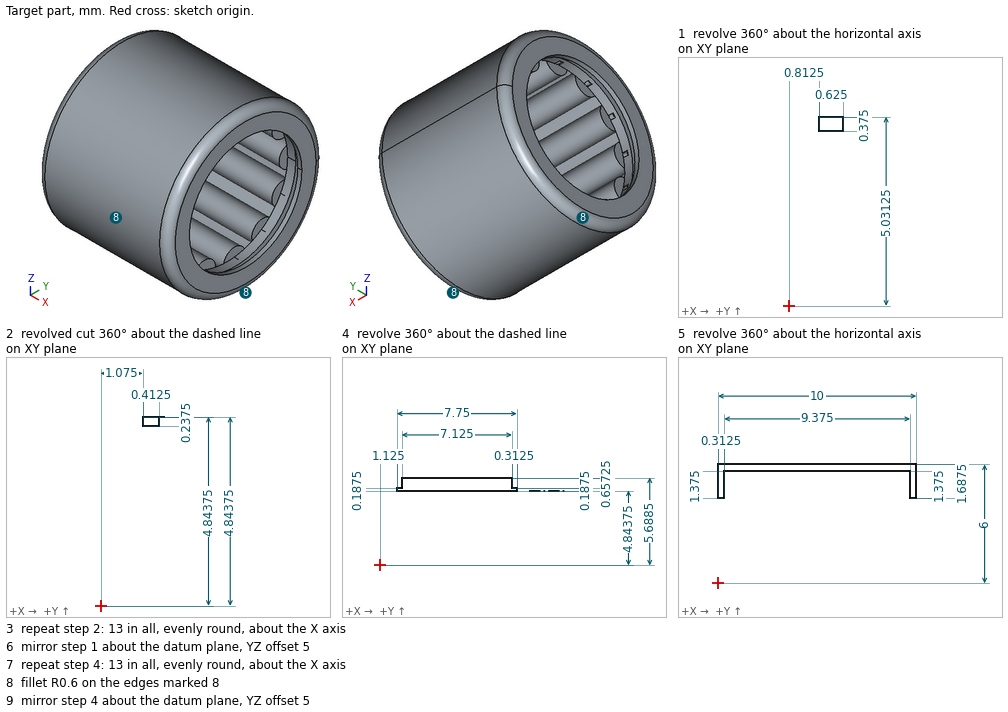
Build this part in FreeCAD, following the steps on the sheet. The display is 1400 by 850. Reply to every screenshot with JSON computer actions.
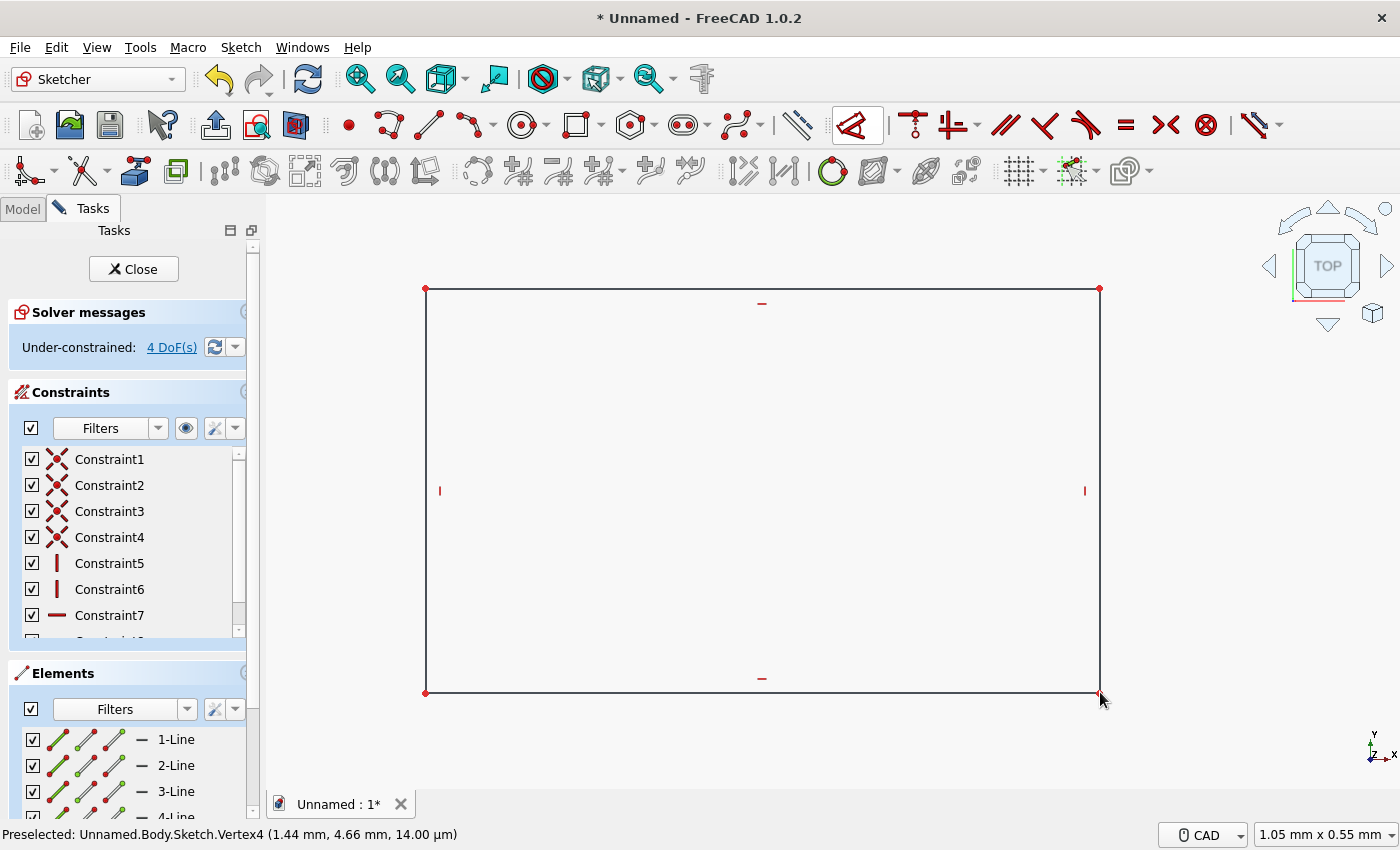
{"action": "key", "text": "d"}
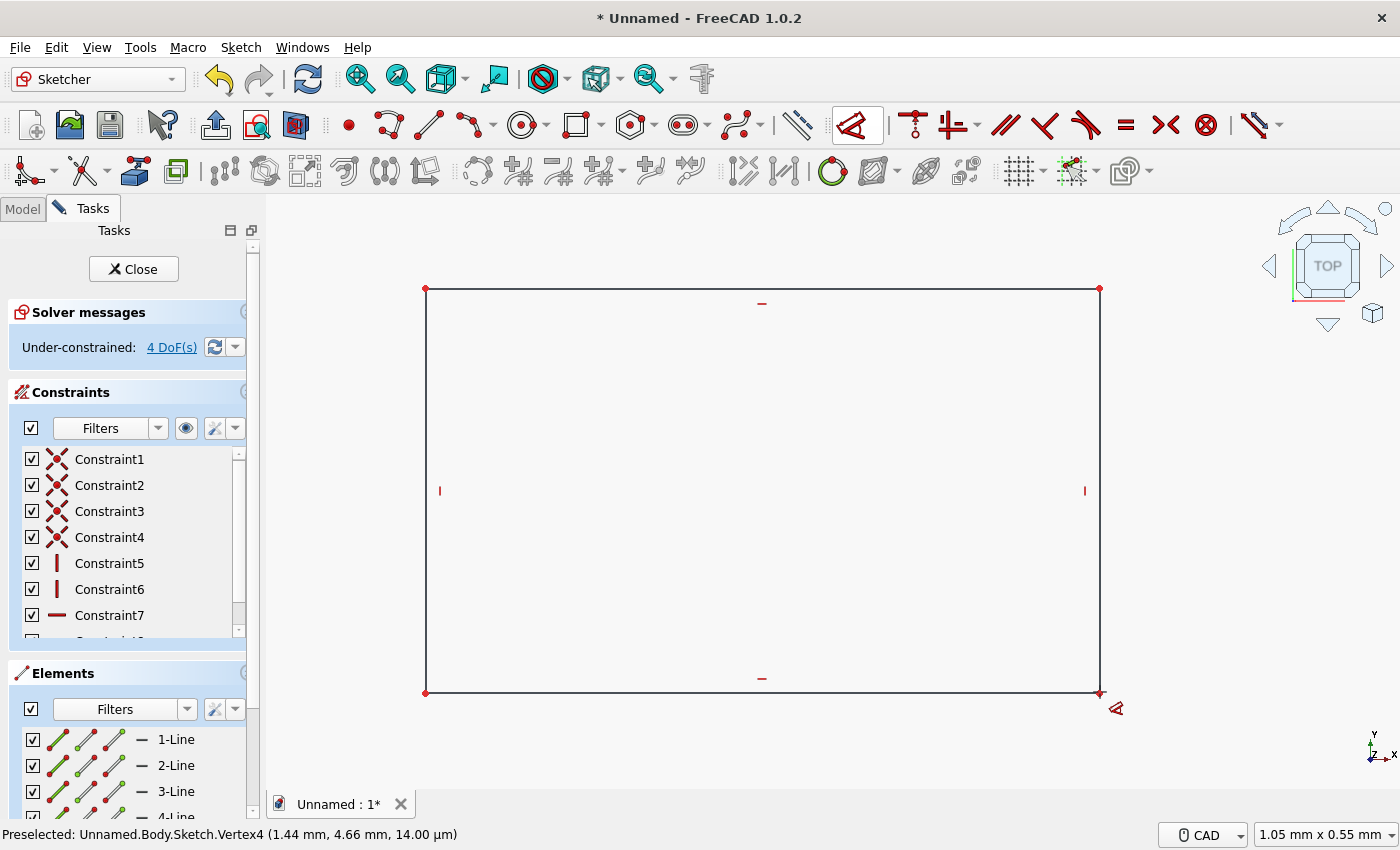
{"action": "left_click", "coordinate": [426, 410]}
{"action": "left_click", "coordinate": [392, 491]}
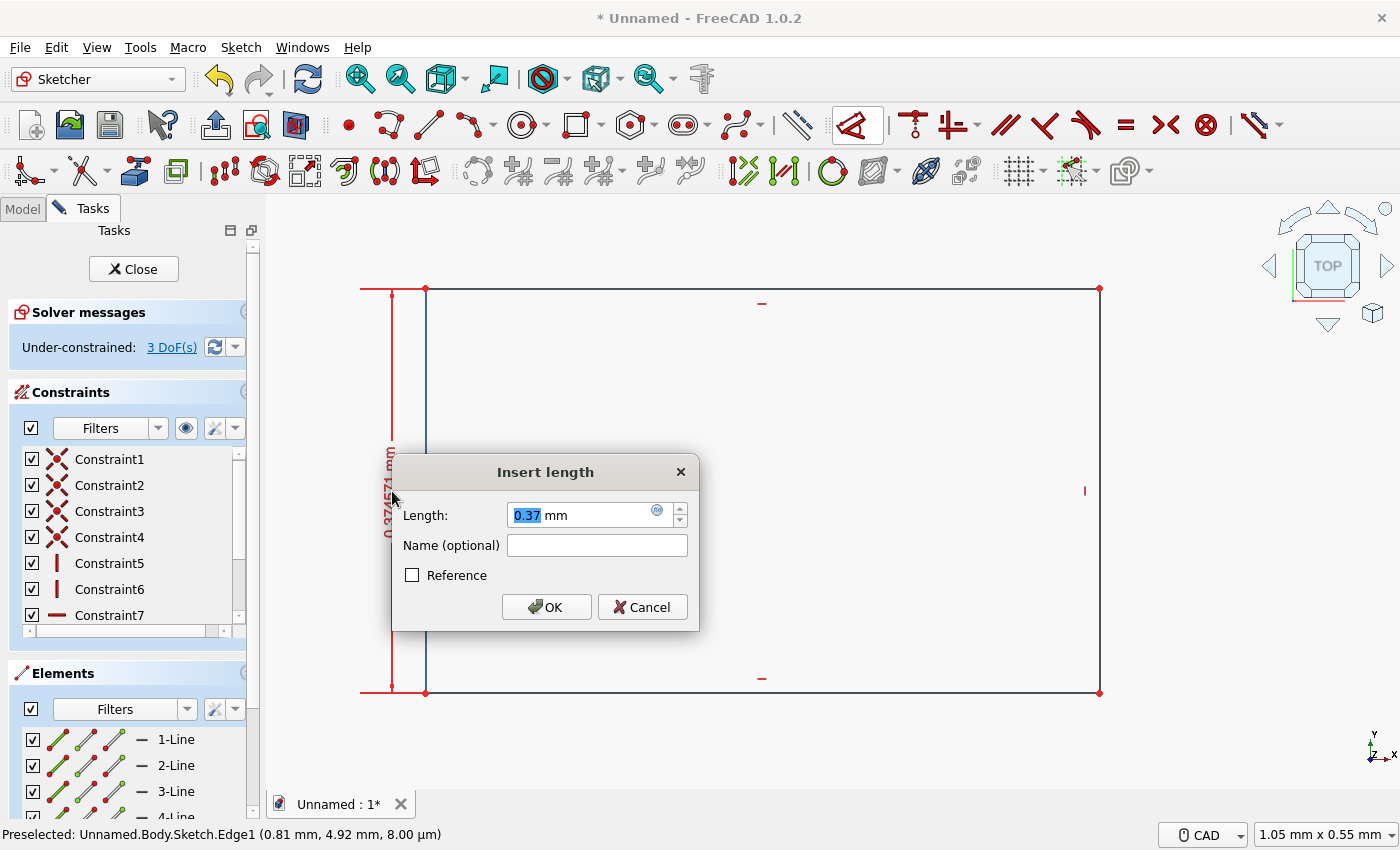
{"action": "type", "text": "0.375"}
{"action": "key", "text": "Return"}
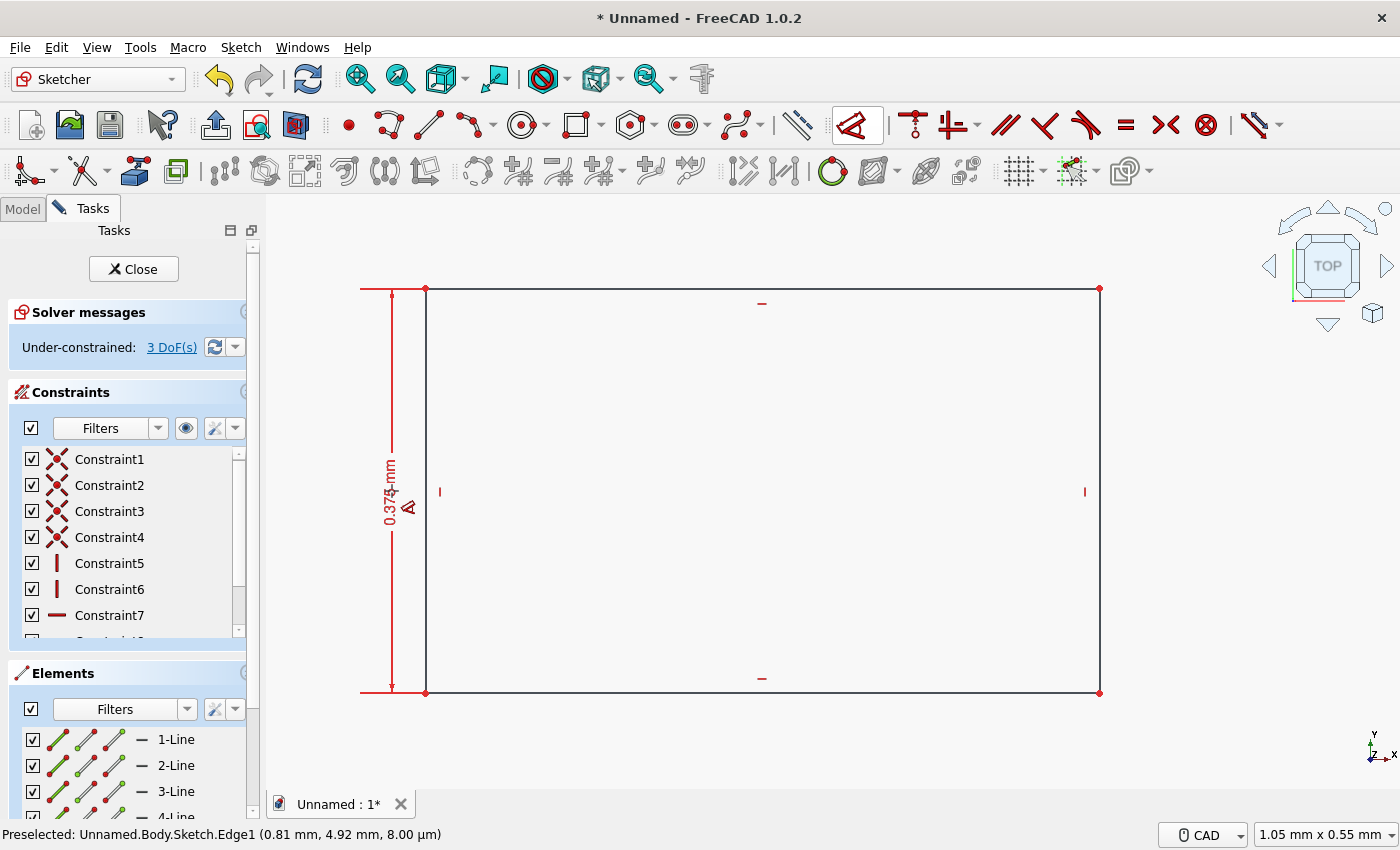
{"action": "left_click", "coordinate": [628, 693]}
{"action": "left_click", "coordinate": [763, 727]}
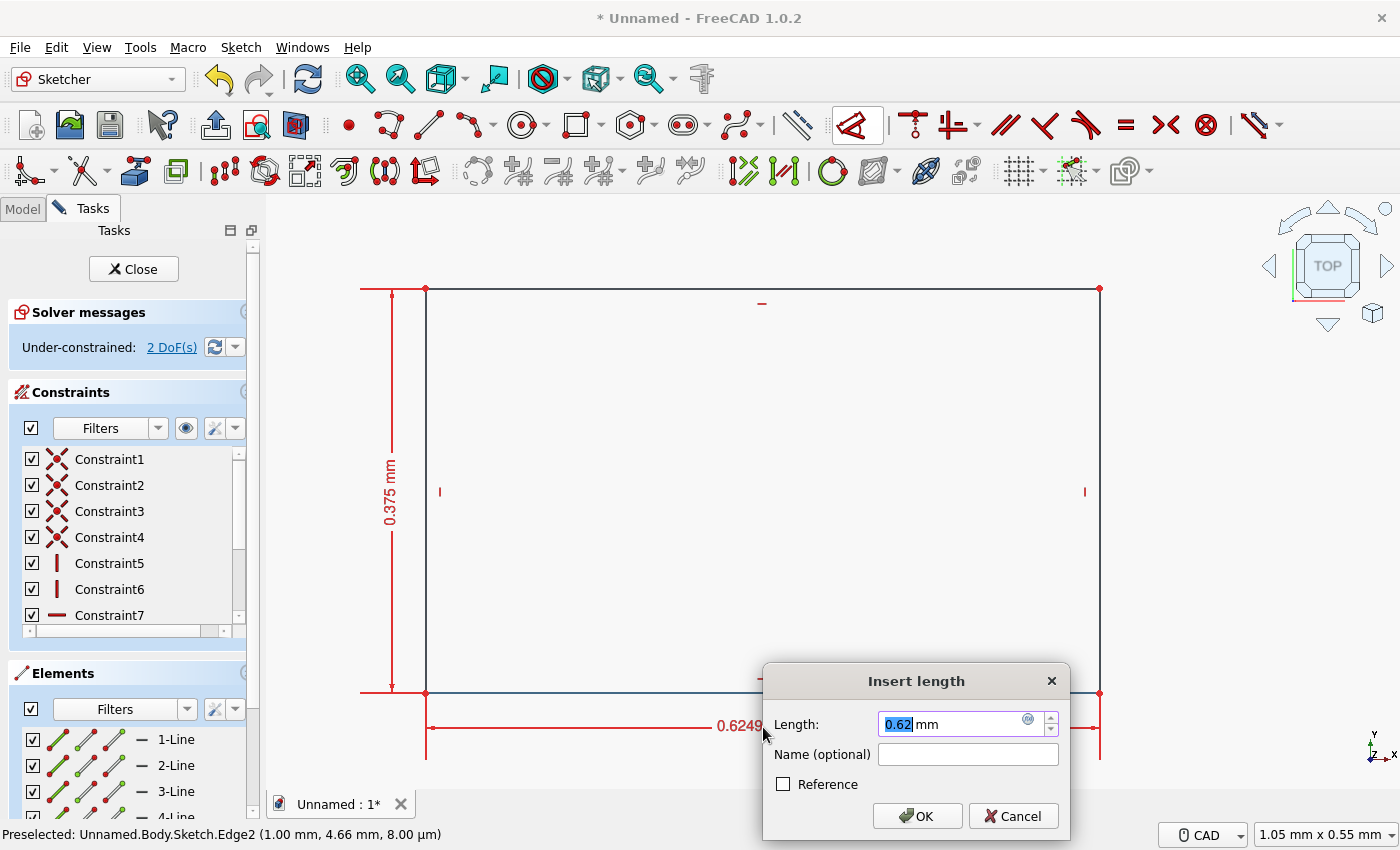
{"action": "type", "text": "0.625"}
{"action": "key", "text": "Return"}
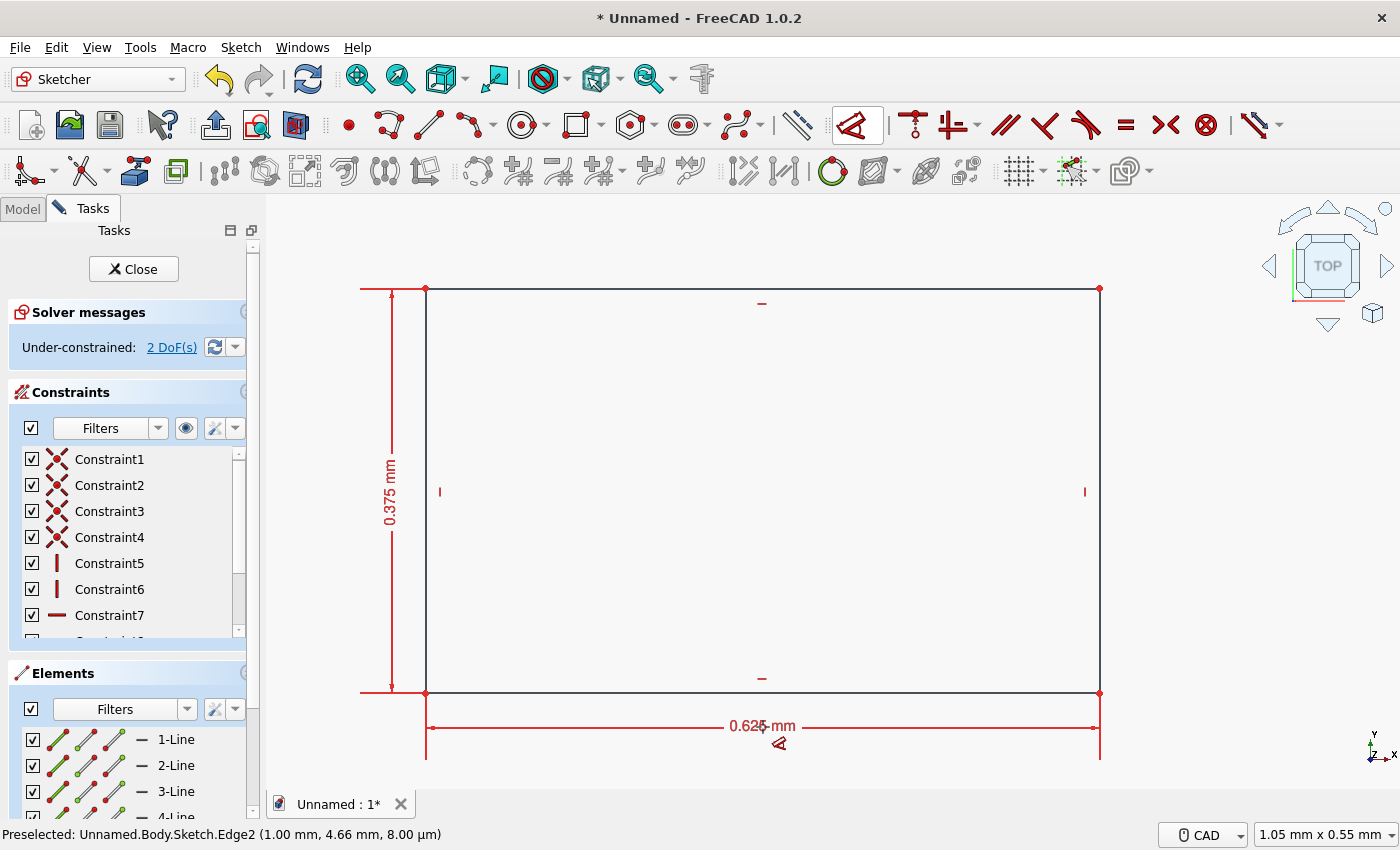
{"action": "left_click", "coordinate": [426, 289]}
{"action": "left_click", "coordinate": [360, 255]}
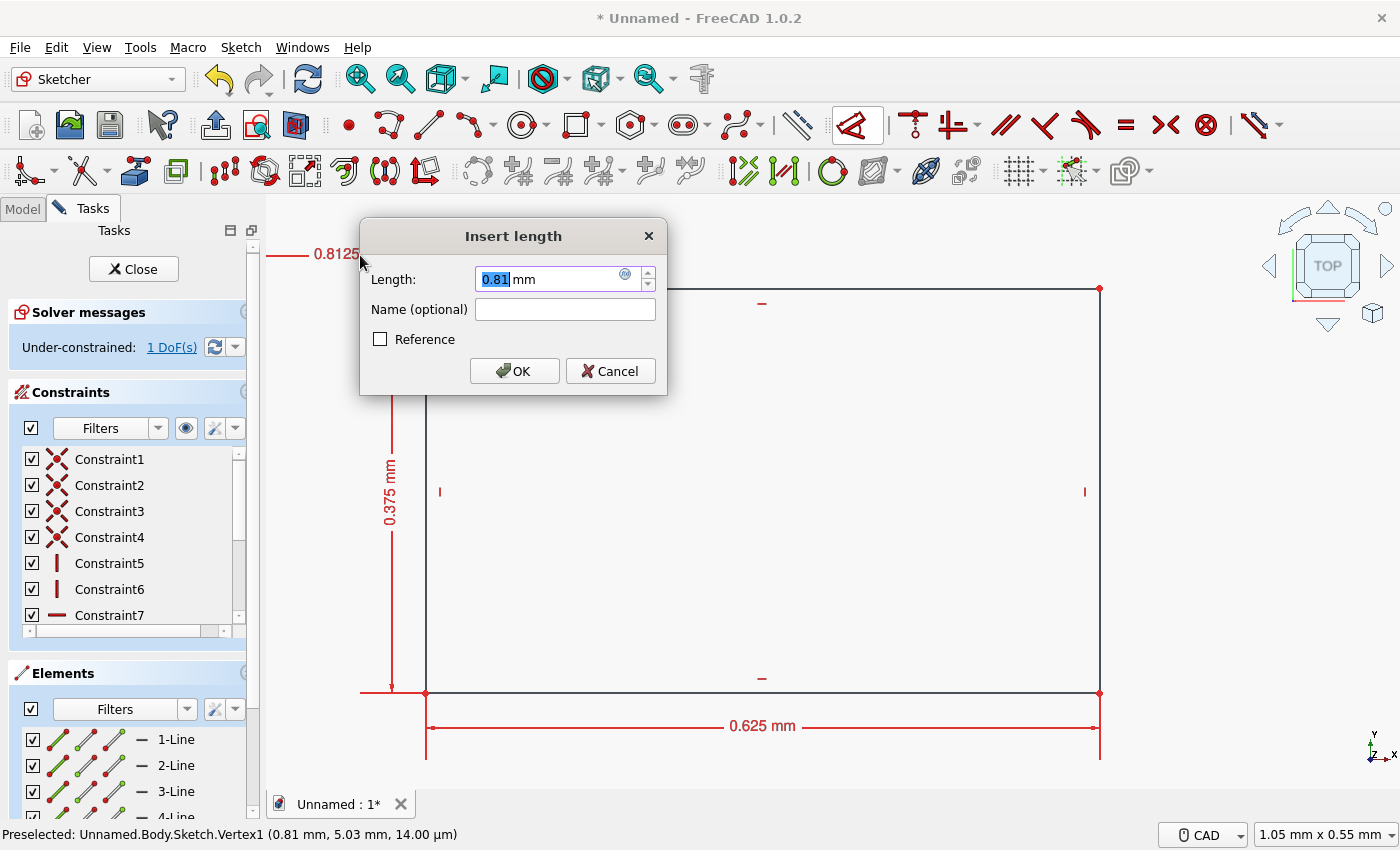
{"action": "type", "text": "0.8125"}
{"action": "key", "text": "Return"}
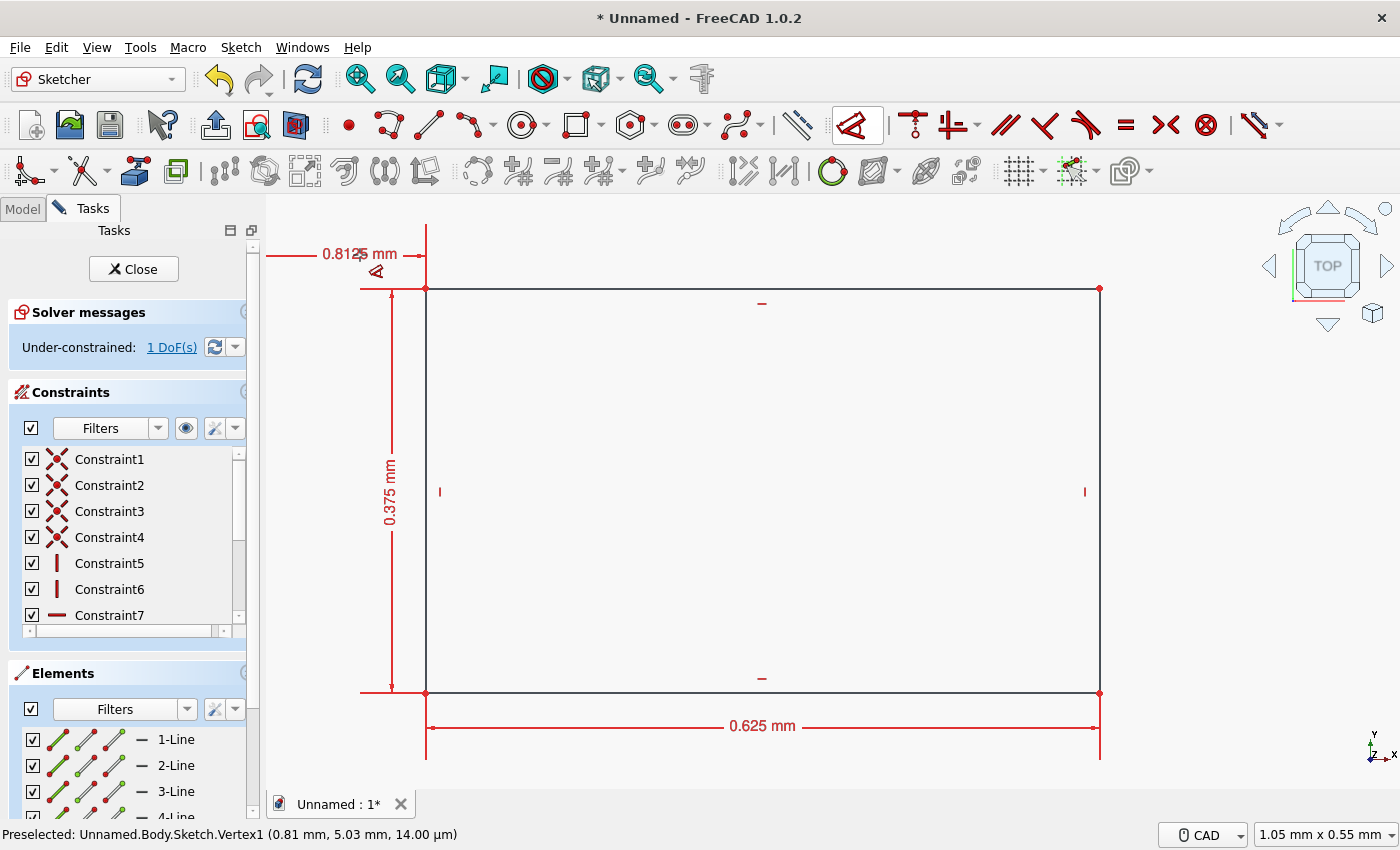
{"action": "left_click", "coordinate": [426, 289]}
{"action": "left_click", "coordinate": [460, 525]}